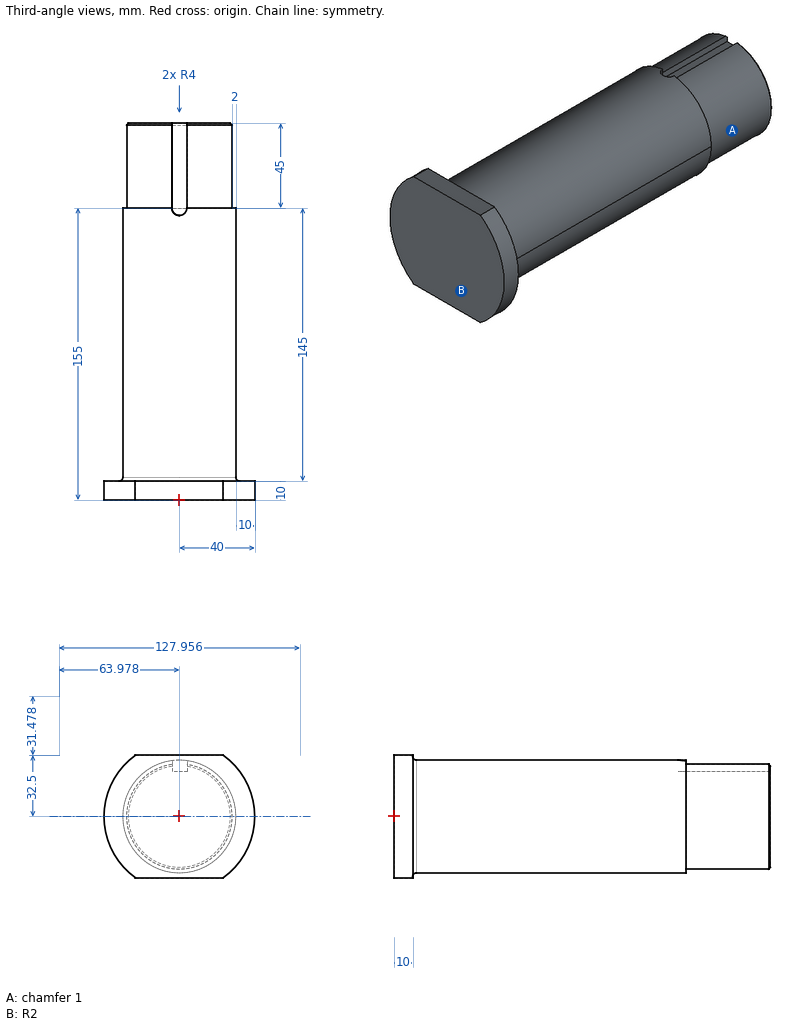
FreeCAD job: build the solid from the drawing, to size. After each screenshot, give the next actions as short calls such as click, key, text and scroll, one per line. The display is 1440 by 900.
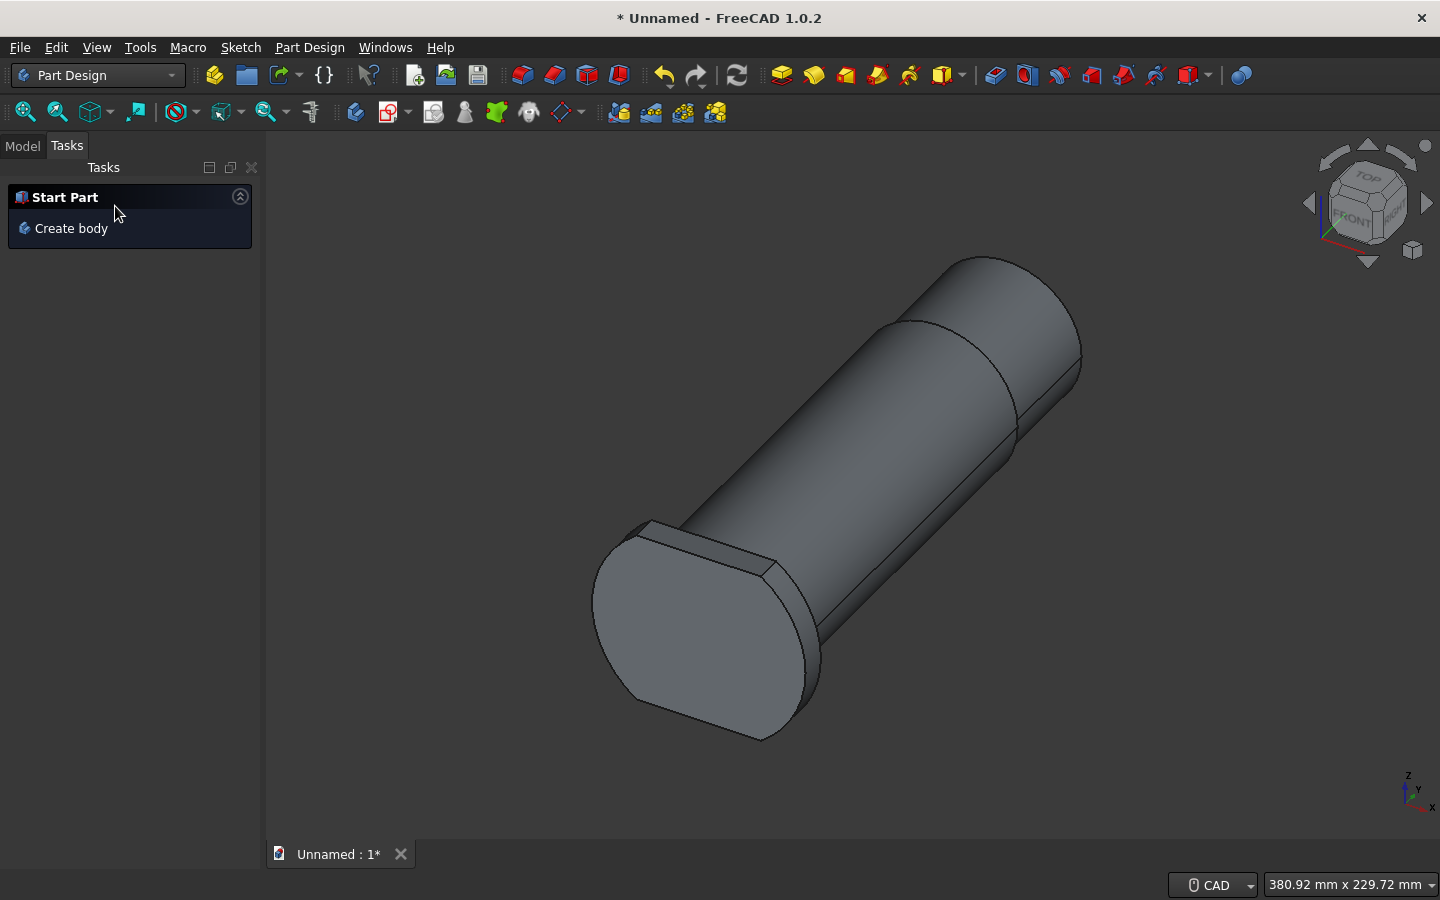
click(23, 145)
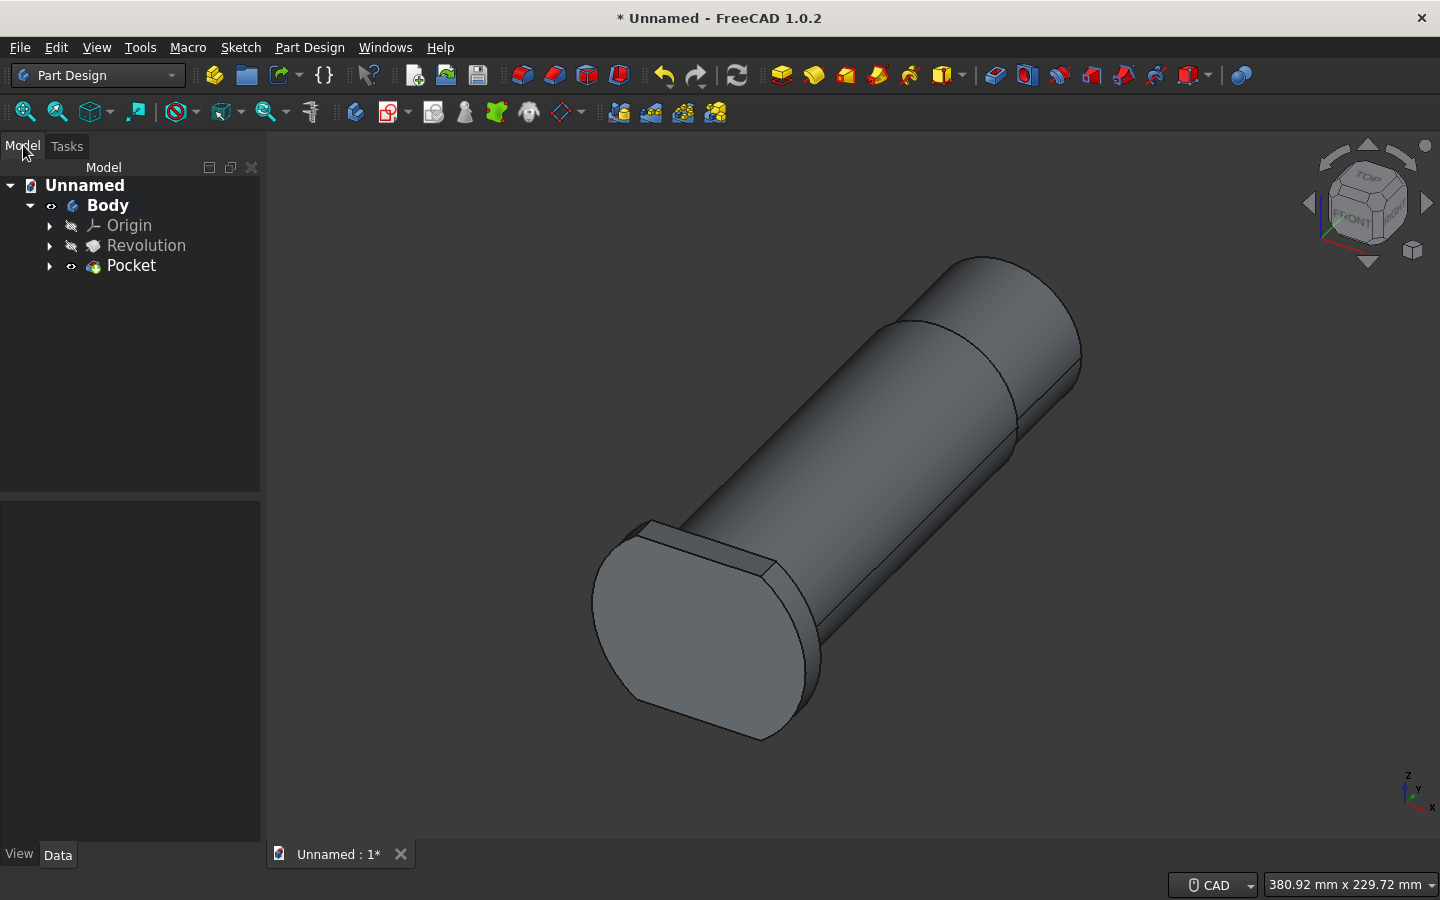
click(50, 226)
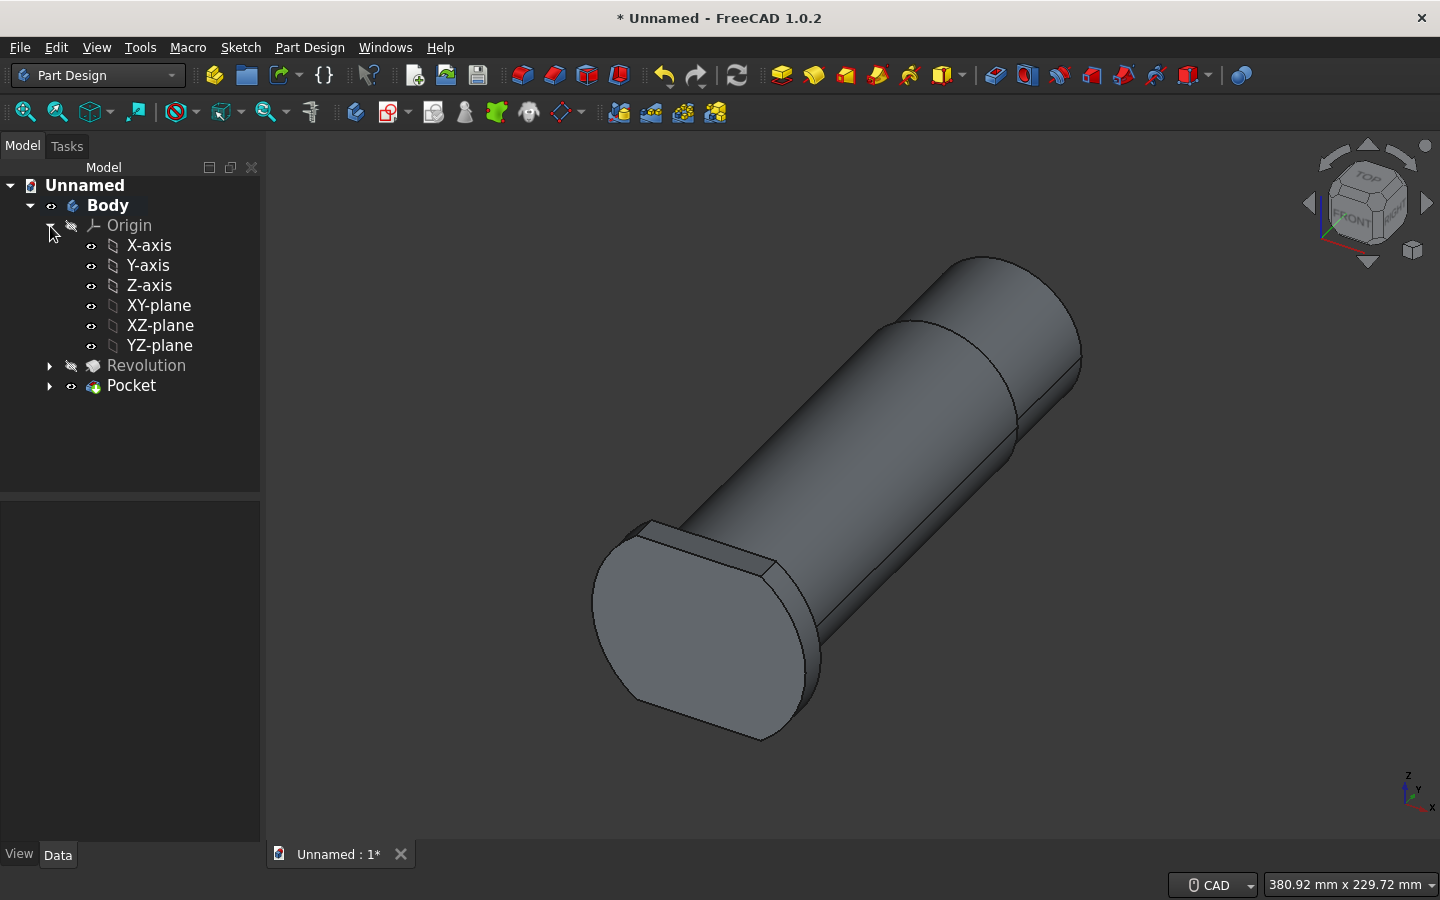
click(136, 306)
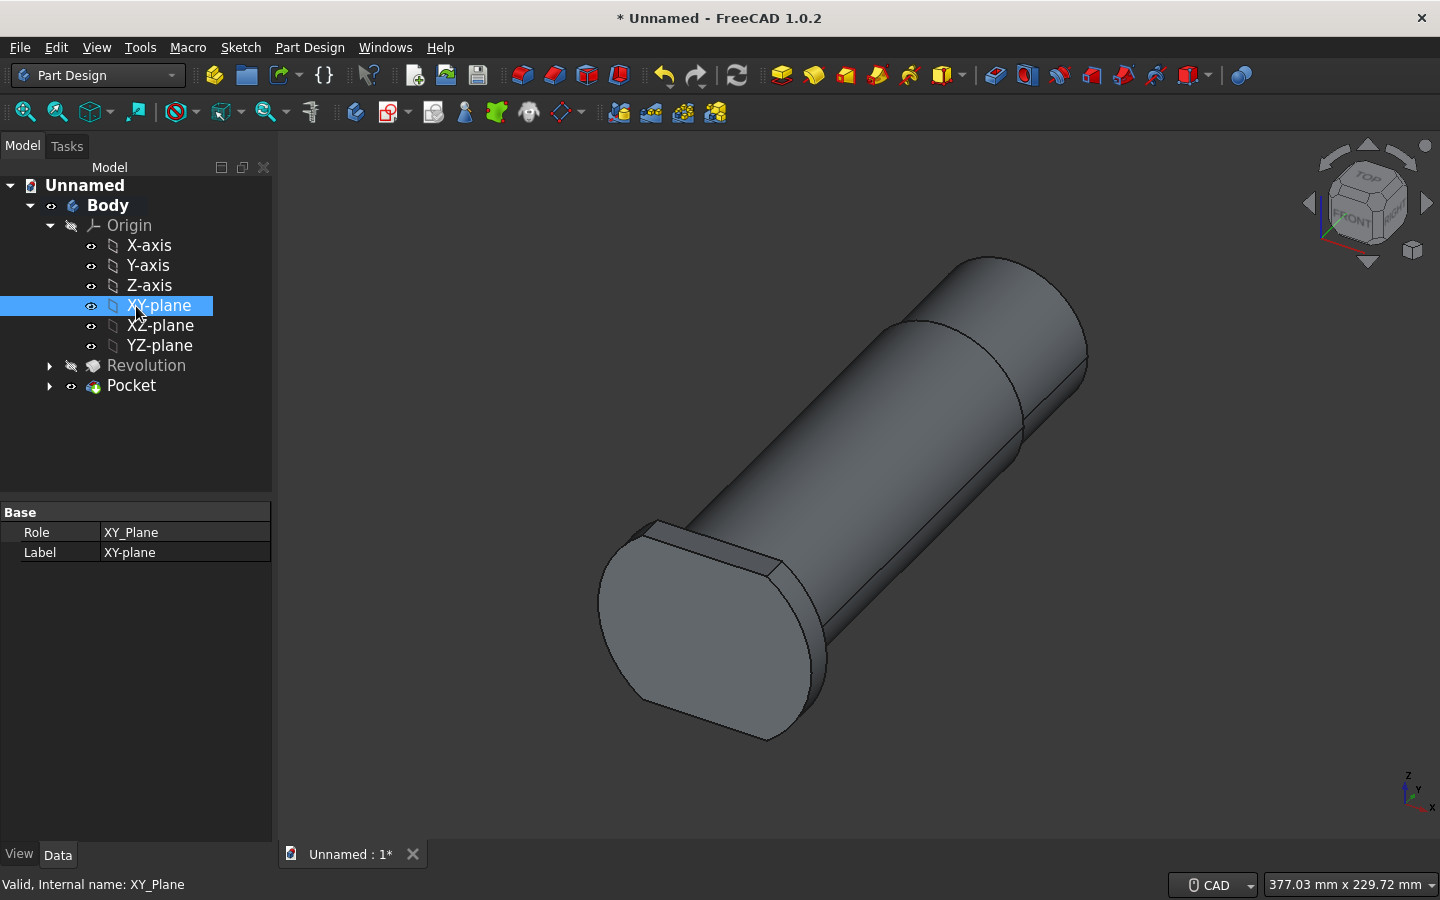
click(562, 112)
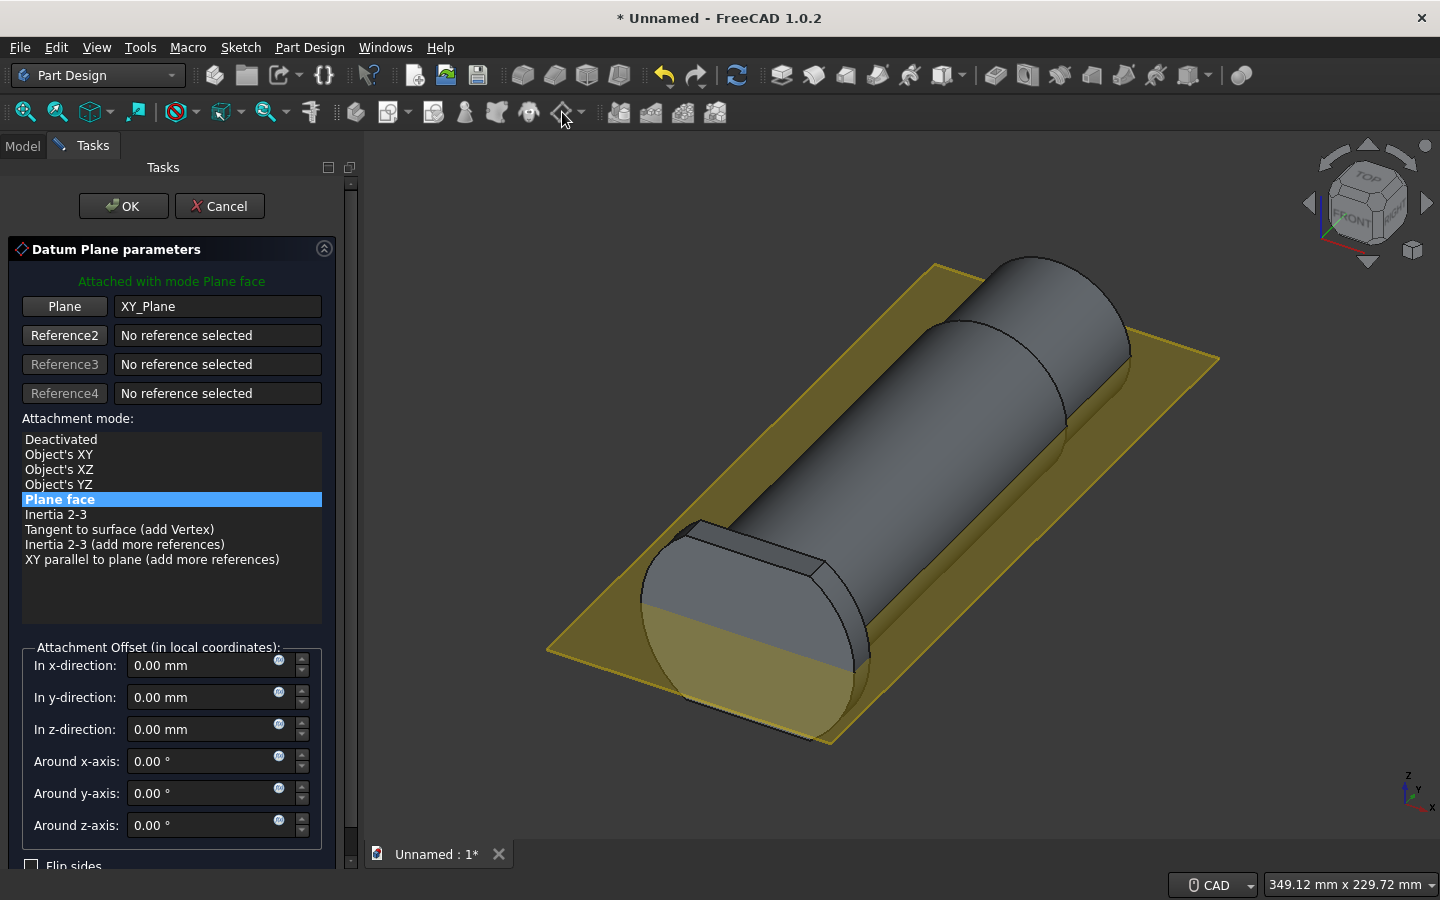
triple_click(210, 729)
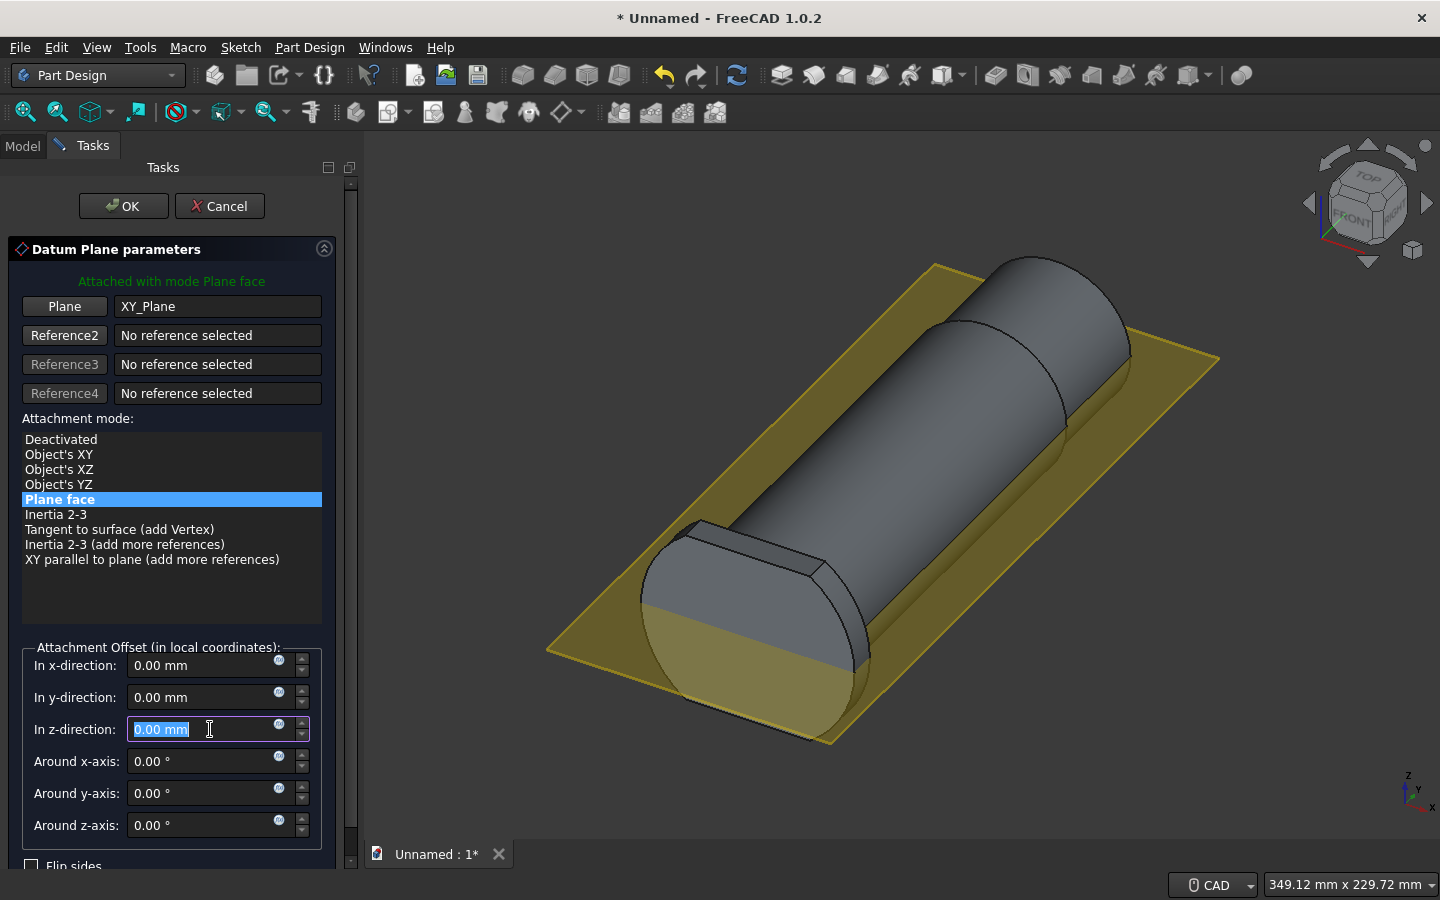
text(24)
key(Tab)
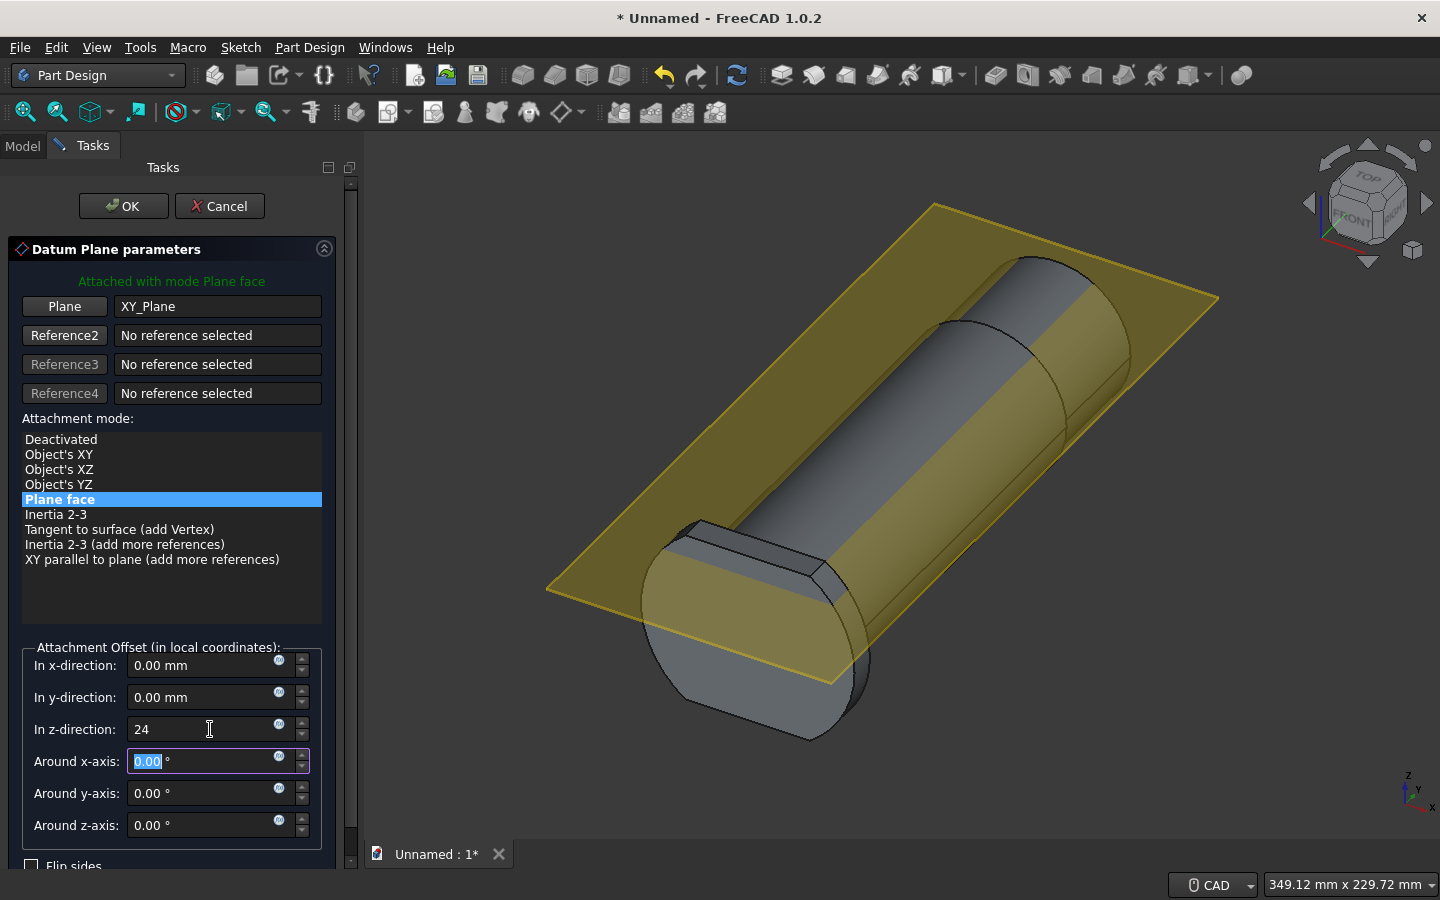
click(124, 206)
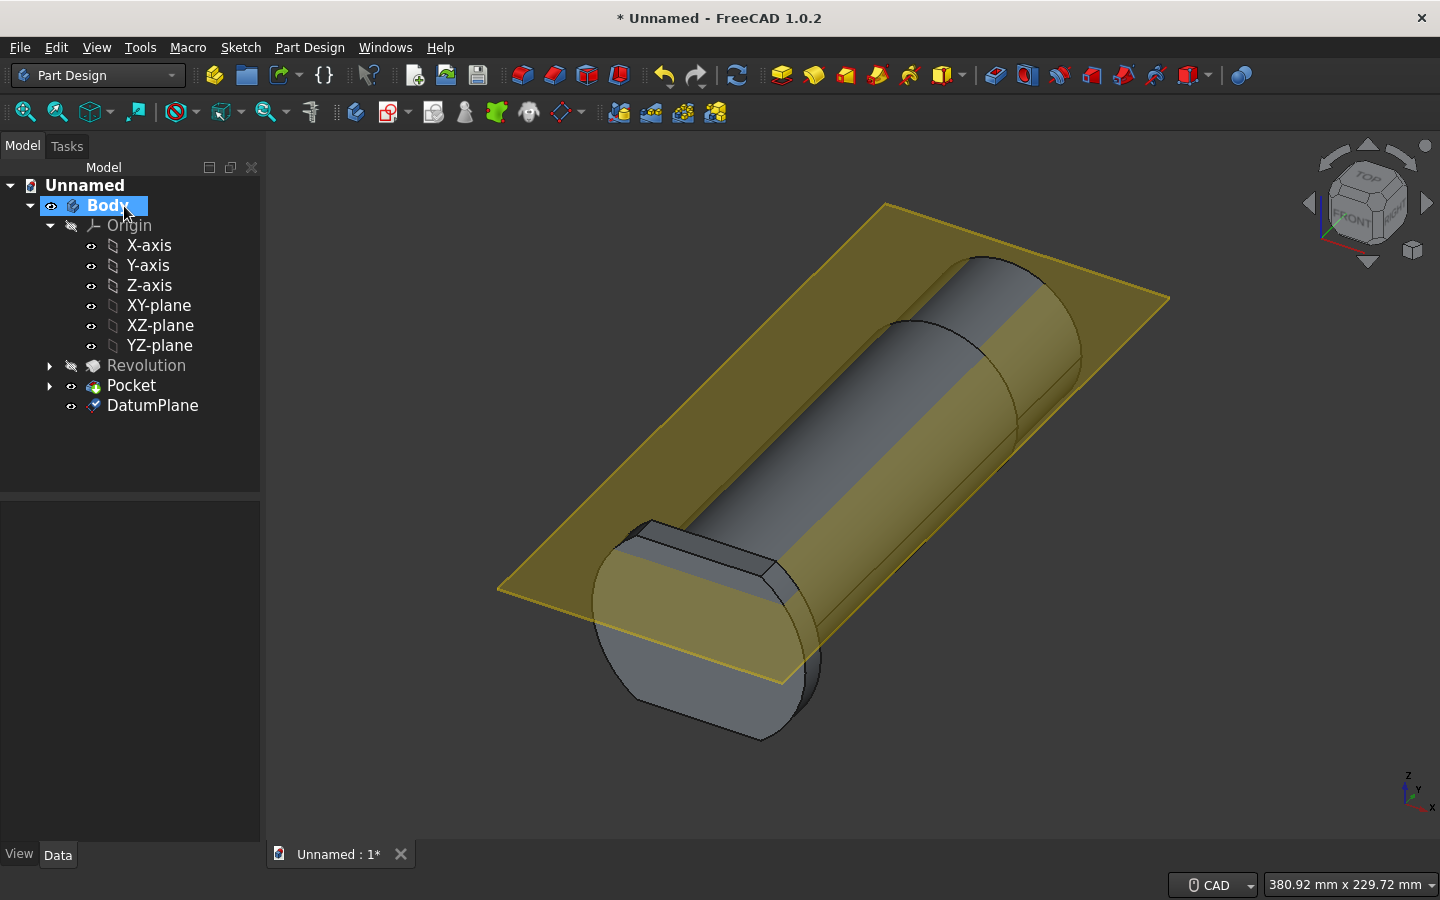
click(116, 406)